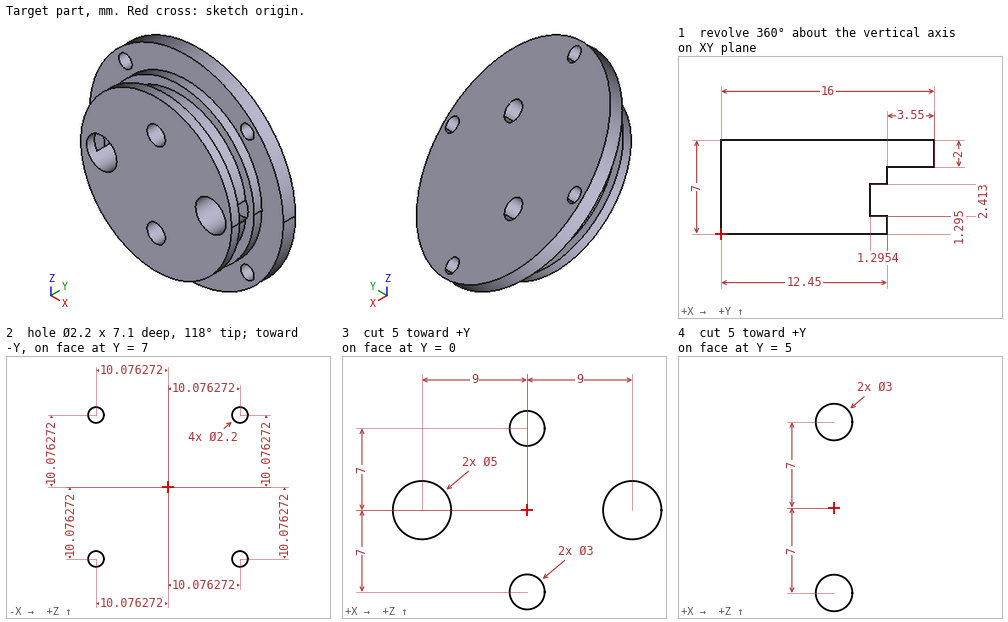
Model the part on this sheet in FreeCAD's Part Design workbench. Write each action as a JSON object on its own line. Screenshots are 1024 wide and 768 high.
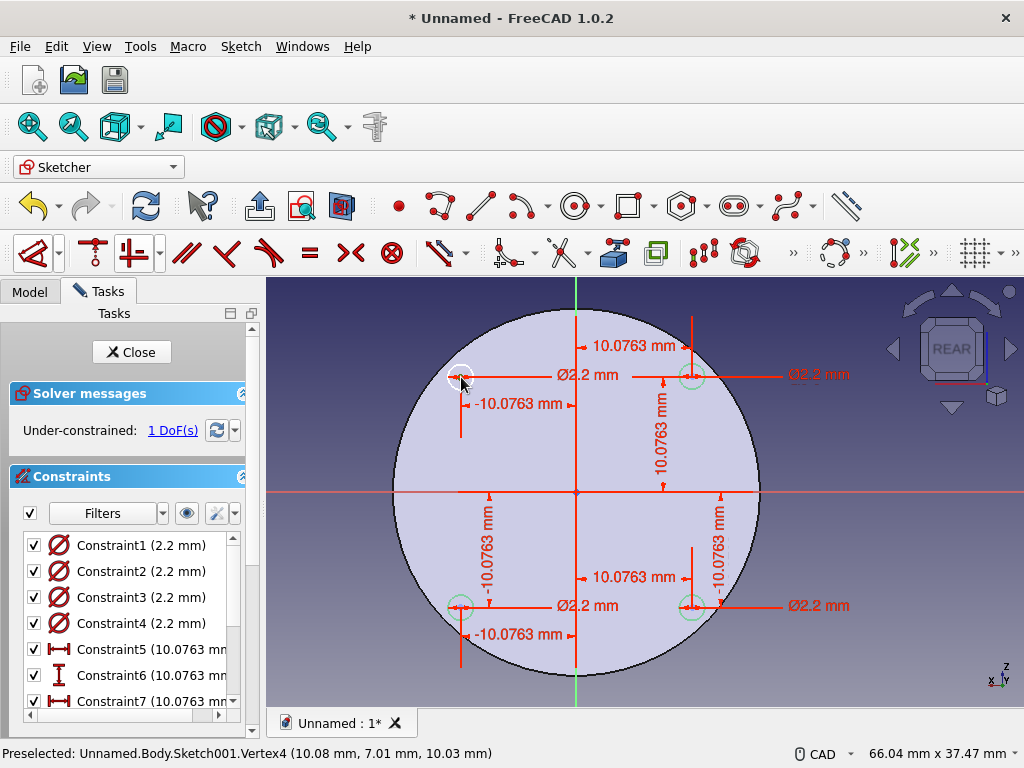
{"action": "left_click", "coordinate": [58, 254]}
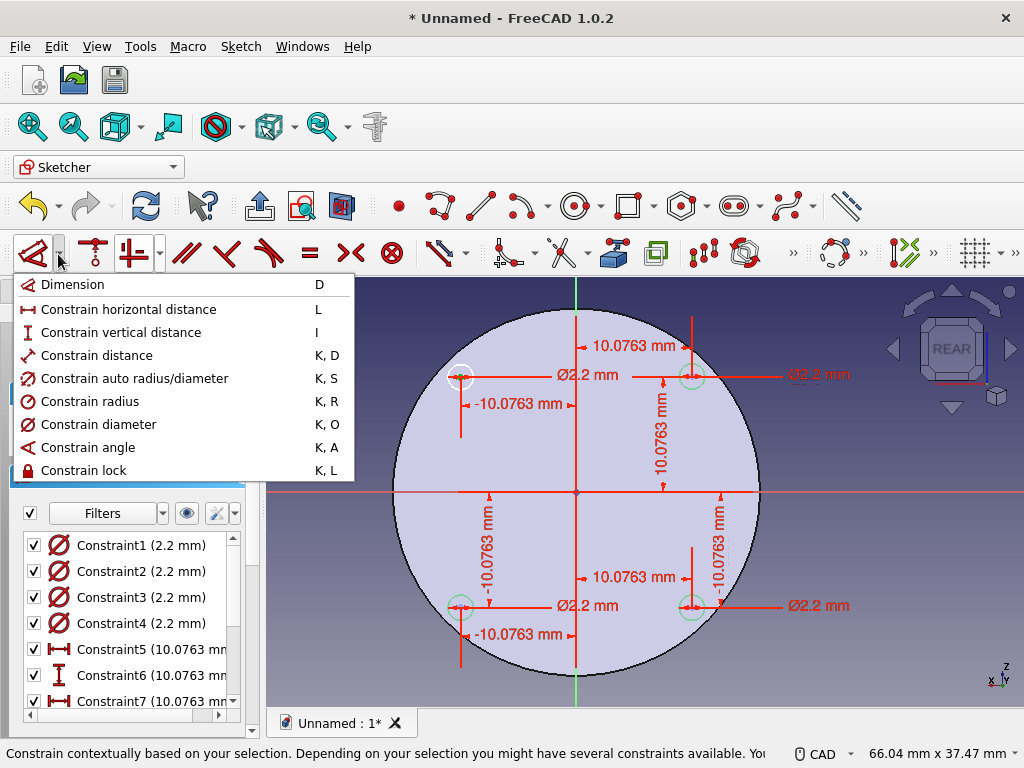
{"action": "left_click", "coordinate": [184, 332]}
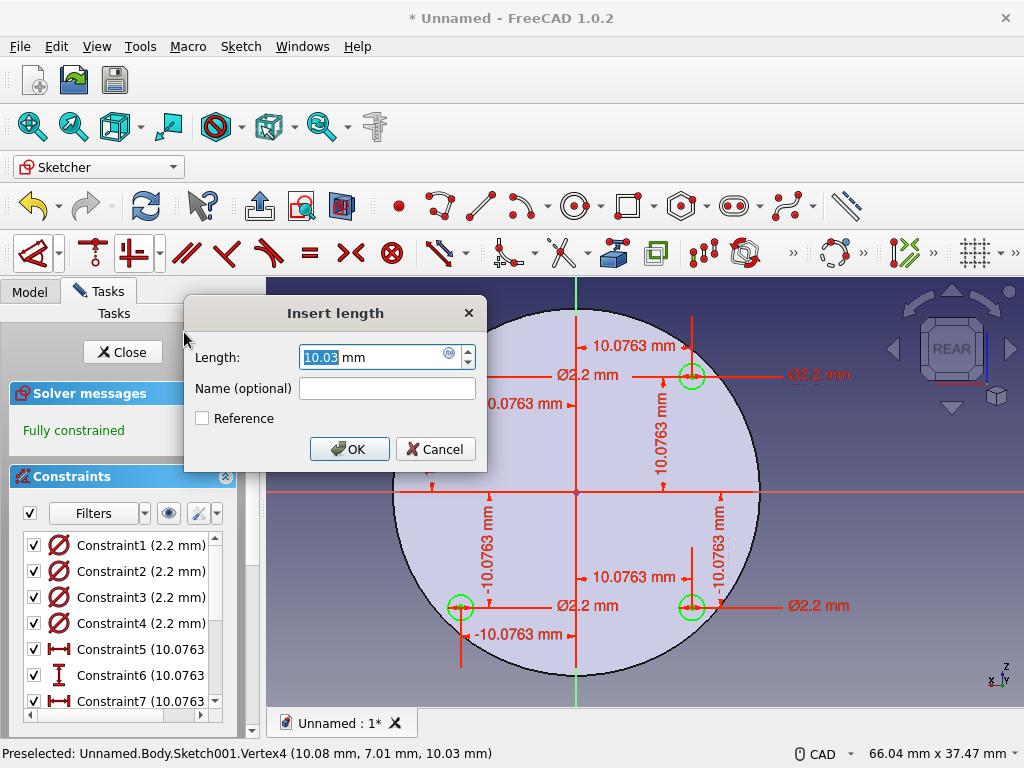
{"action": "type", "text": "10.076272"}
{"action": "key", "text": "Return"}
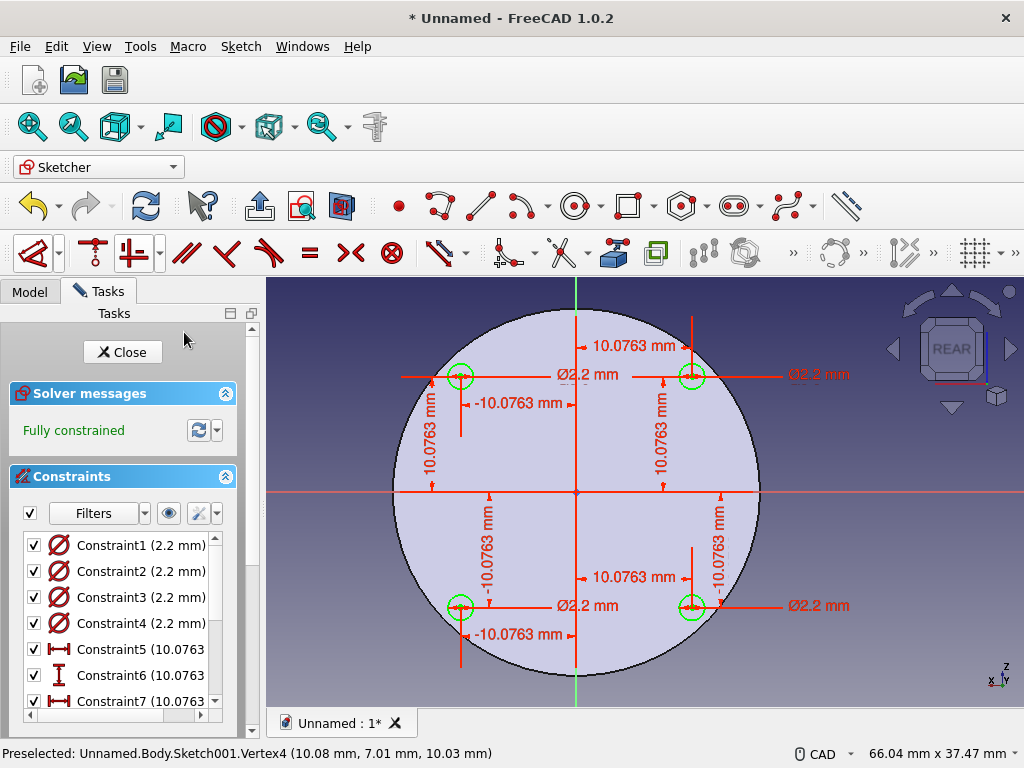
{"action": "left_click", "coordinate": [123, 352]}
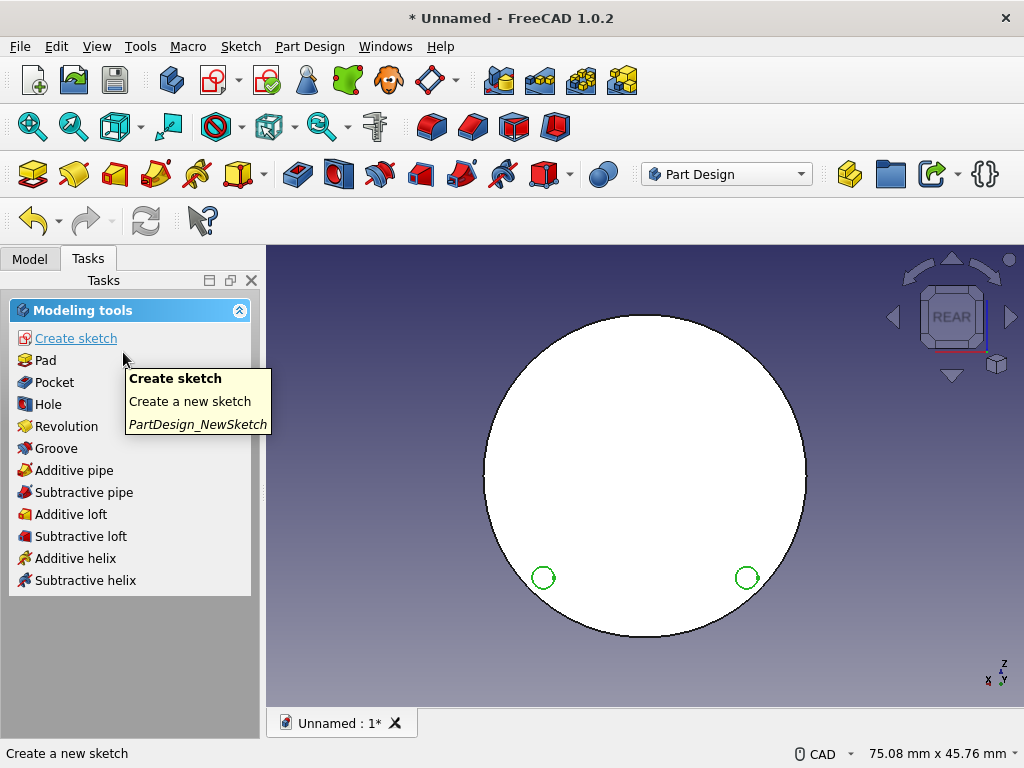
{"action": "left_click", "coordinate": [339, 174]}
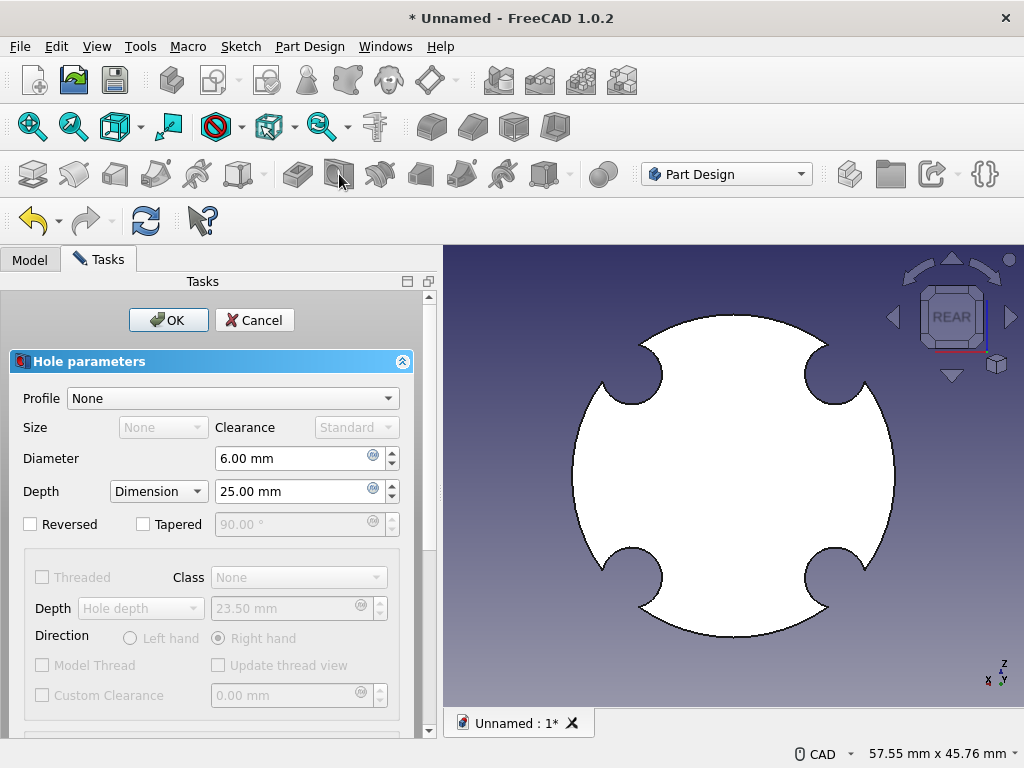
{"action": "triple_click", "coordinate": [300, 458]}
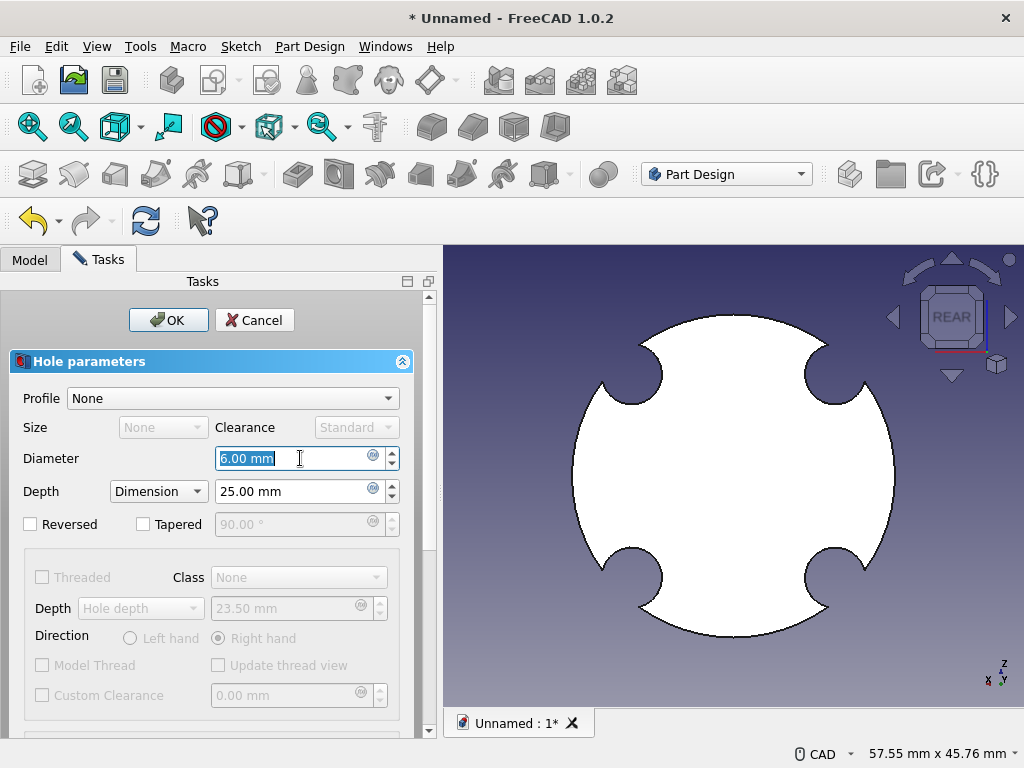
{"action": "type", "text": "2.2"}
{"action": "key", "text": "Tab"}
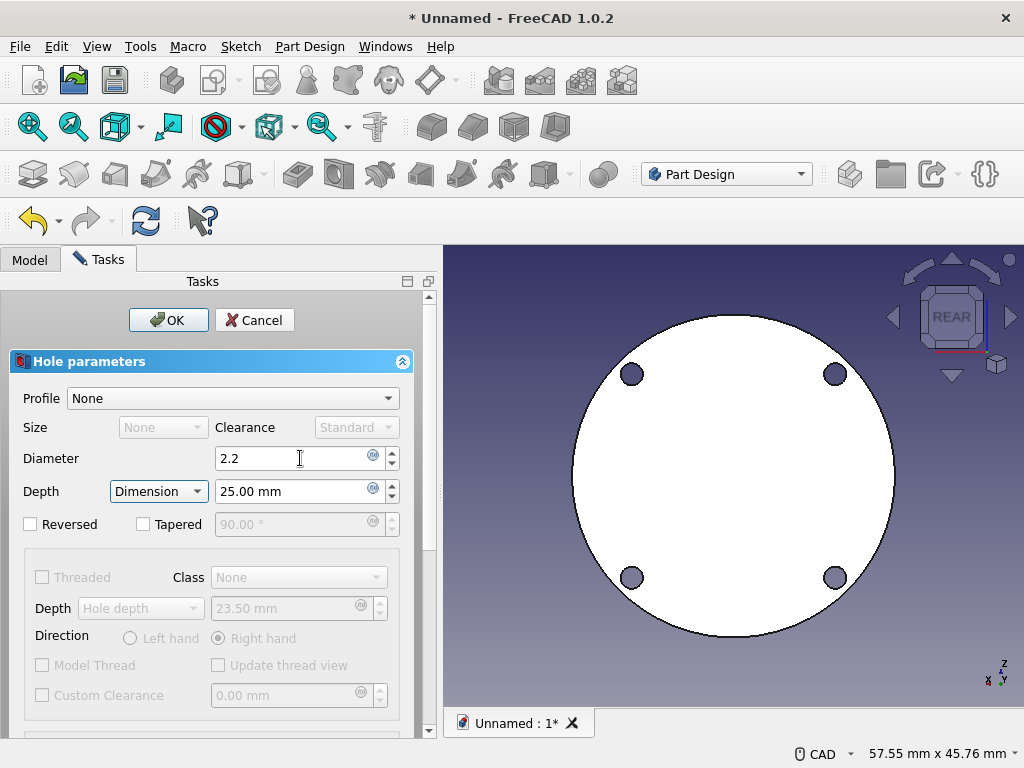
{"action": "triple_click", "coordinate": [300, 492]}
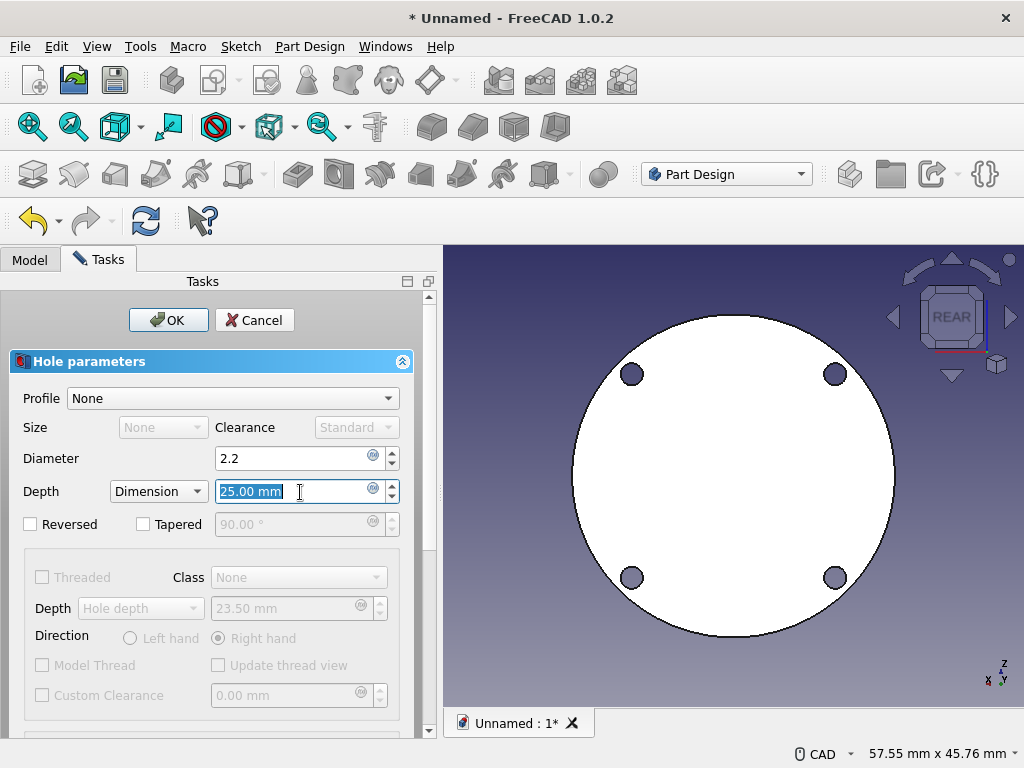
{"action": "type", "text": "7.1"}
{"action": "key", "text": "Tab"}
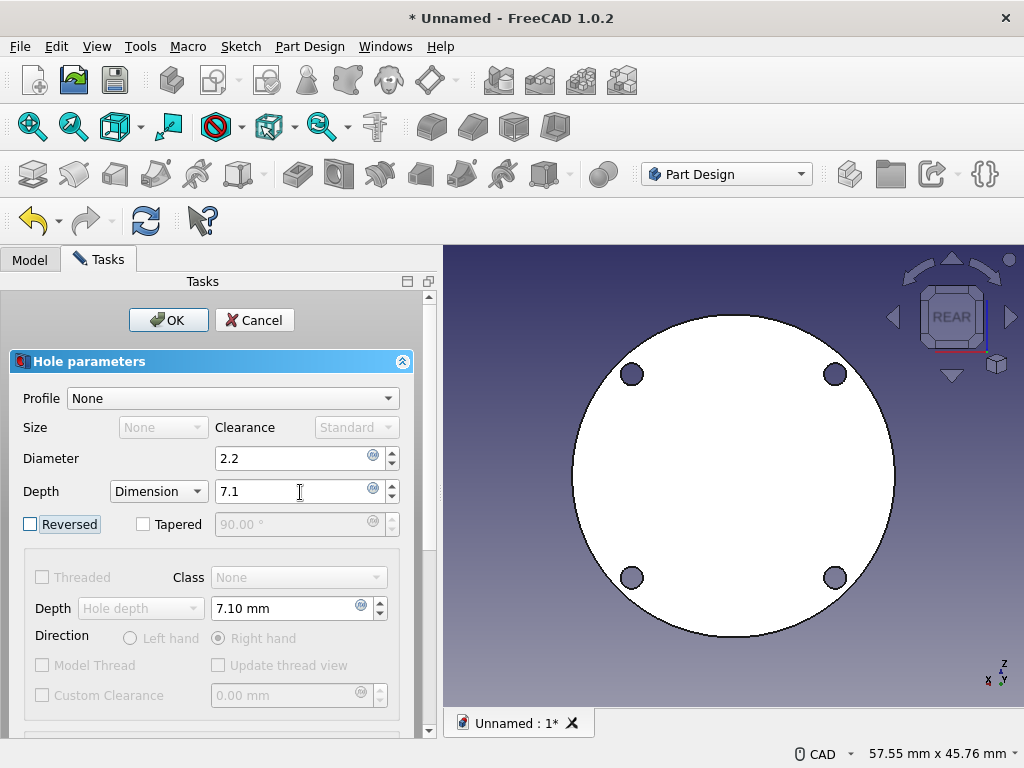
{"action": "left_click", "coordinate": [169, 320]}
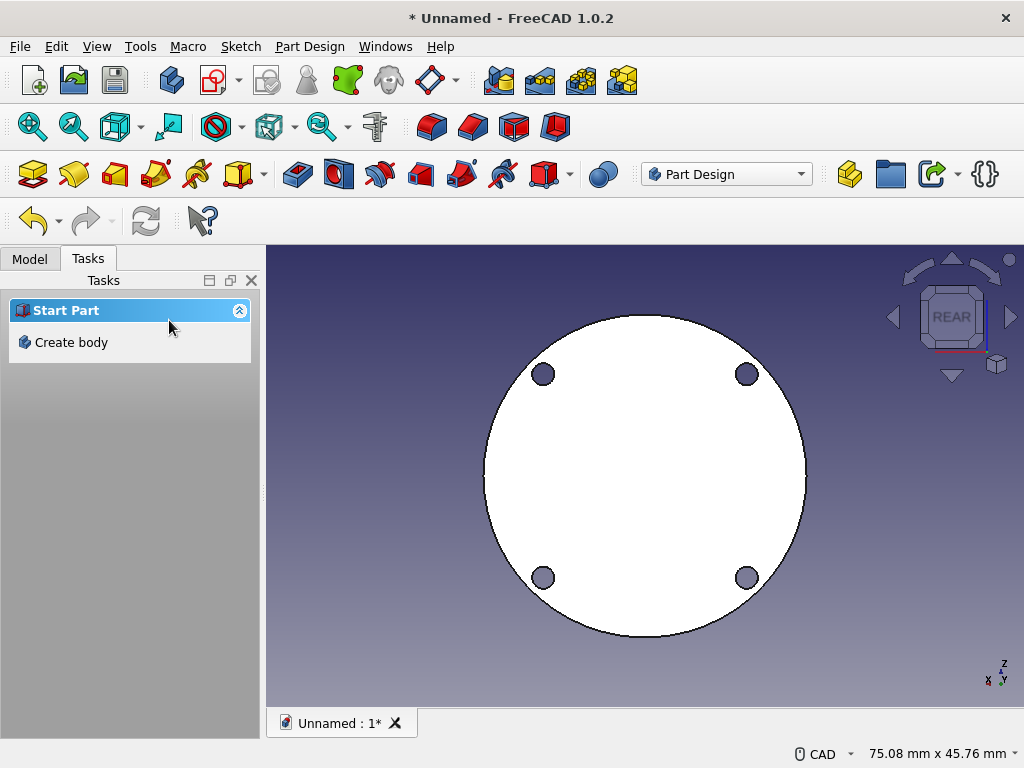
{"action": "key", "text": "0"}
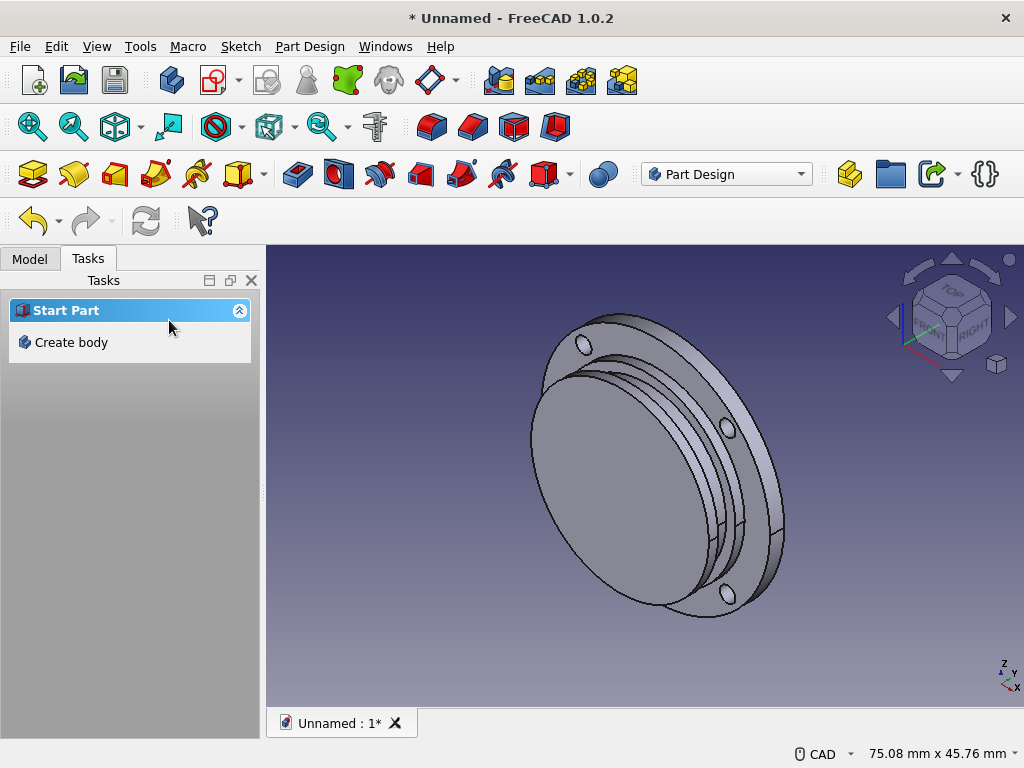
{"action": "left_click", "coordinate": [620, 489]}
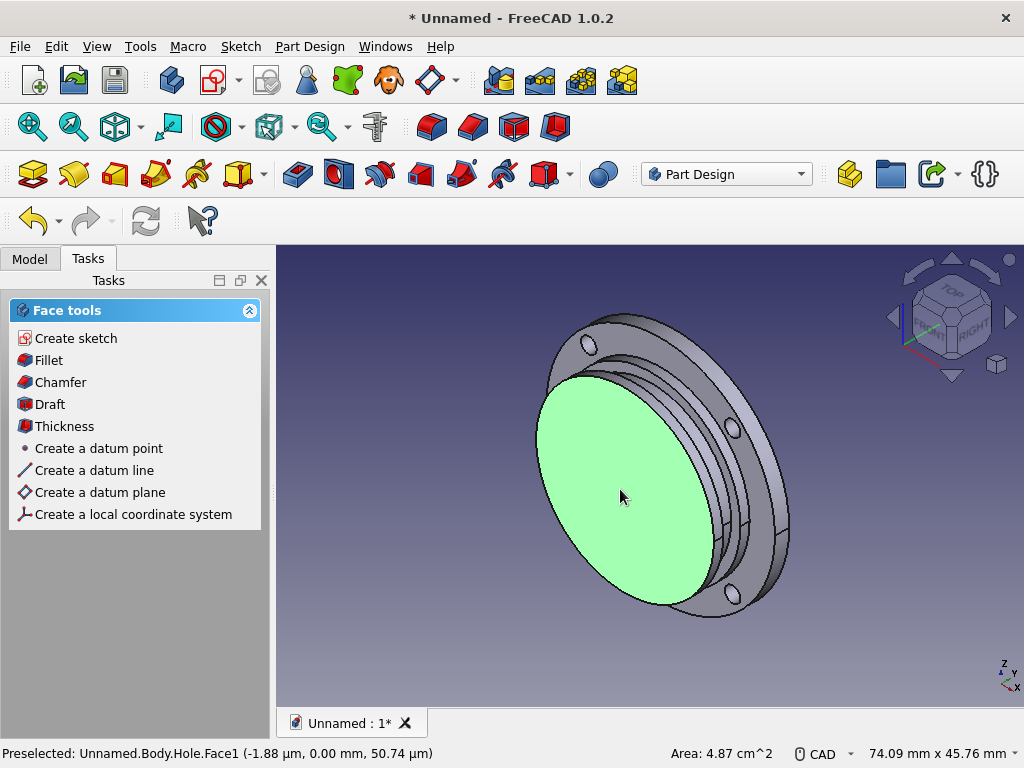
{"action": "left_click", "coordinate": [212, 80]}